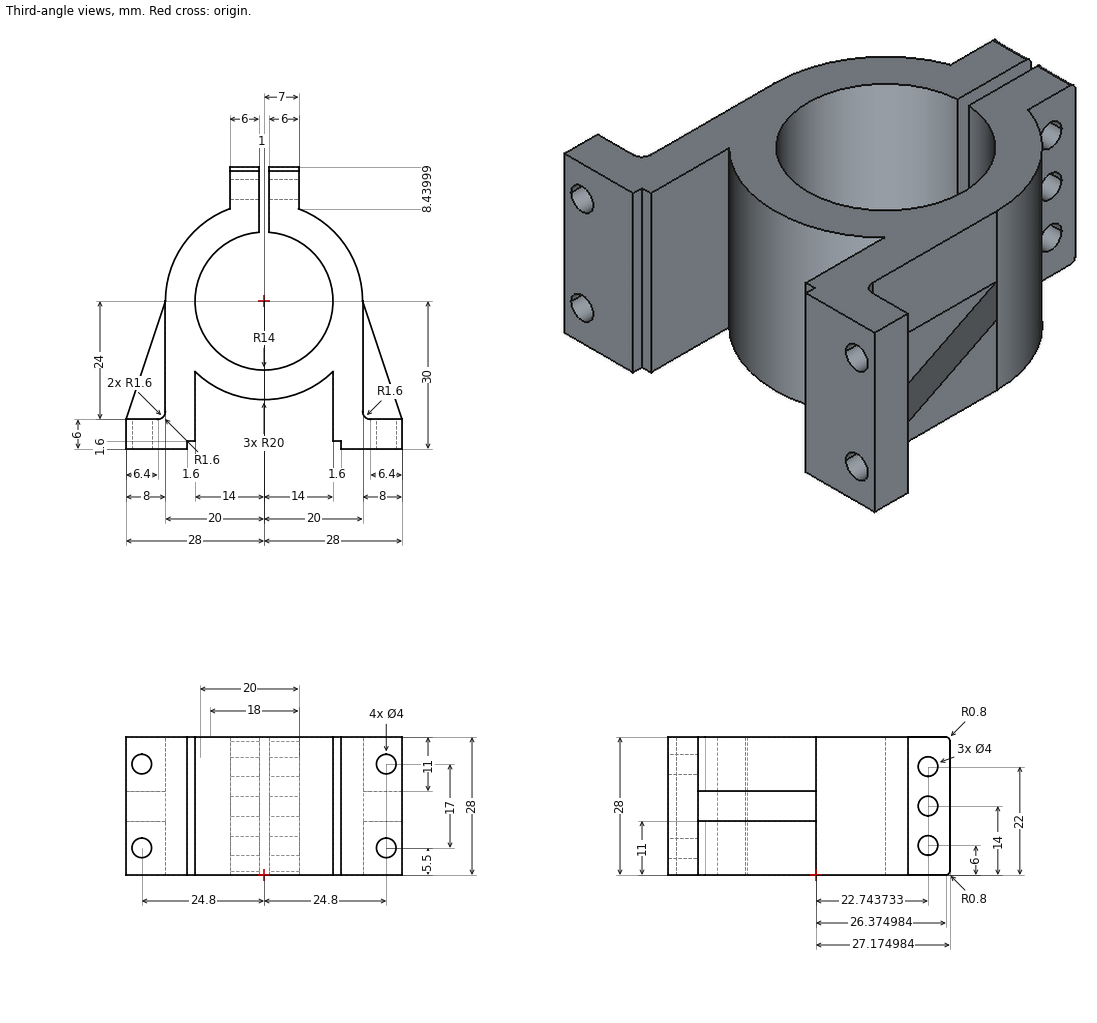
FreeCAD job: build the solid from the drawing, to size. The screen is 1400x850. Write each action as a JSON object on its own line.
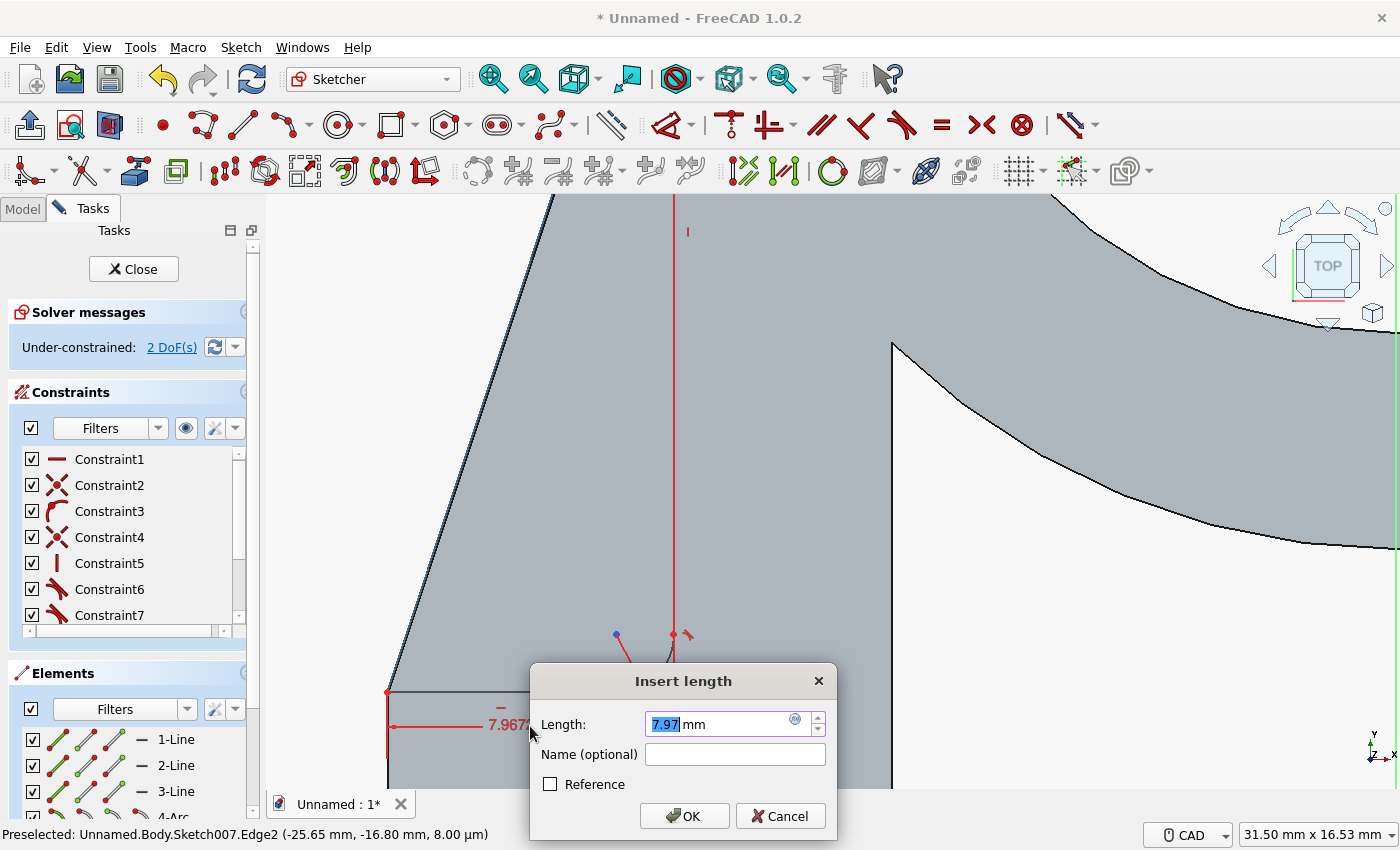
{"action": "type", "text": "8"}
{"action": "key", "text": "Return"}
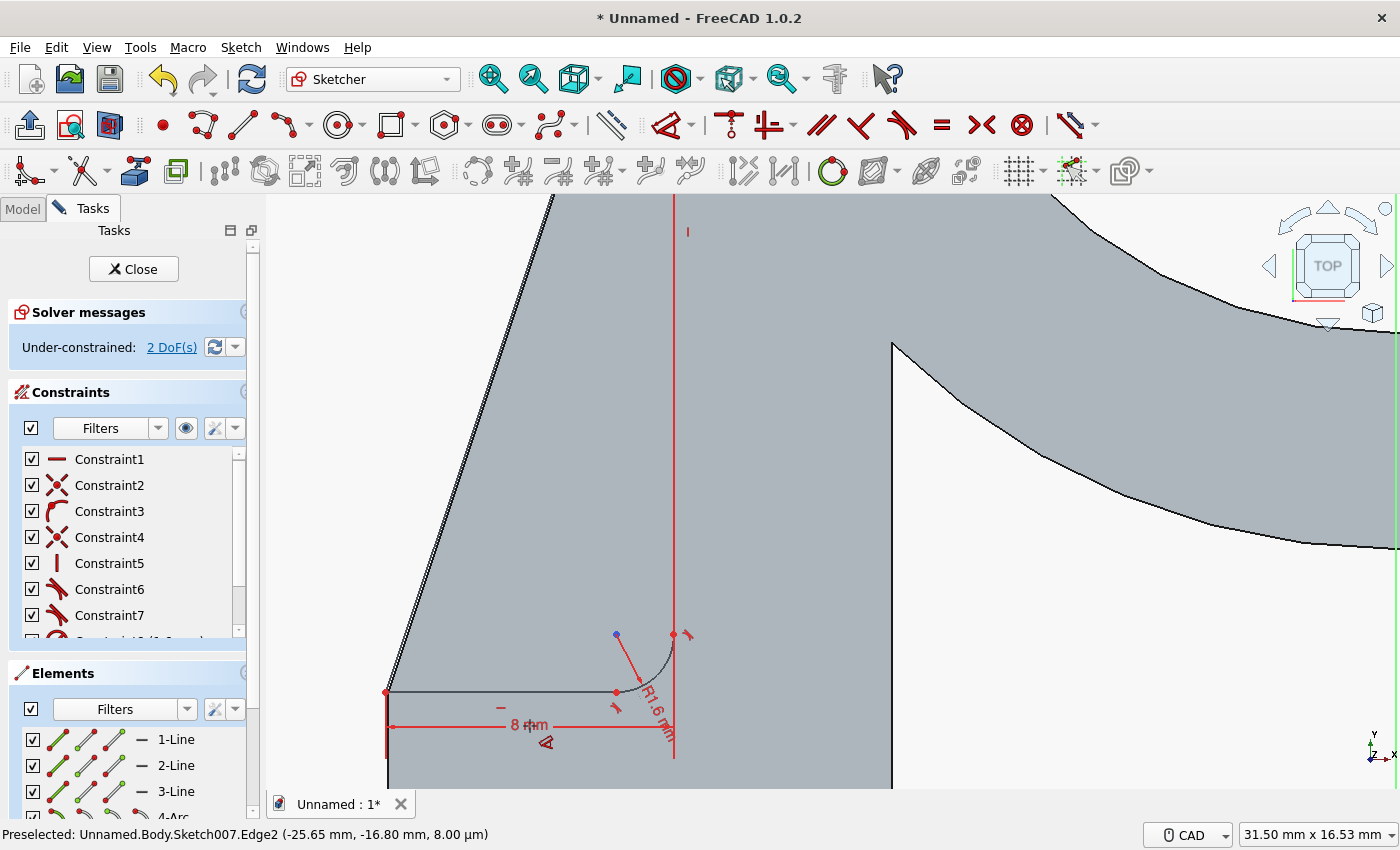
{"action": "left_click", "coordinate": [616, 692]}
{"action": "left_click", "coordinate": [582, 457]}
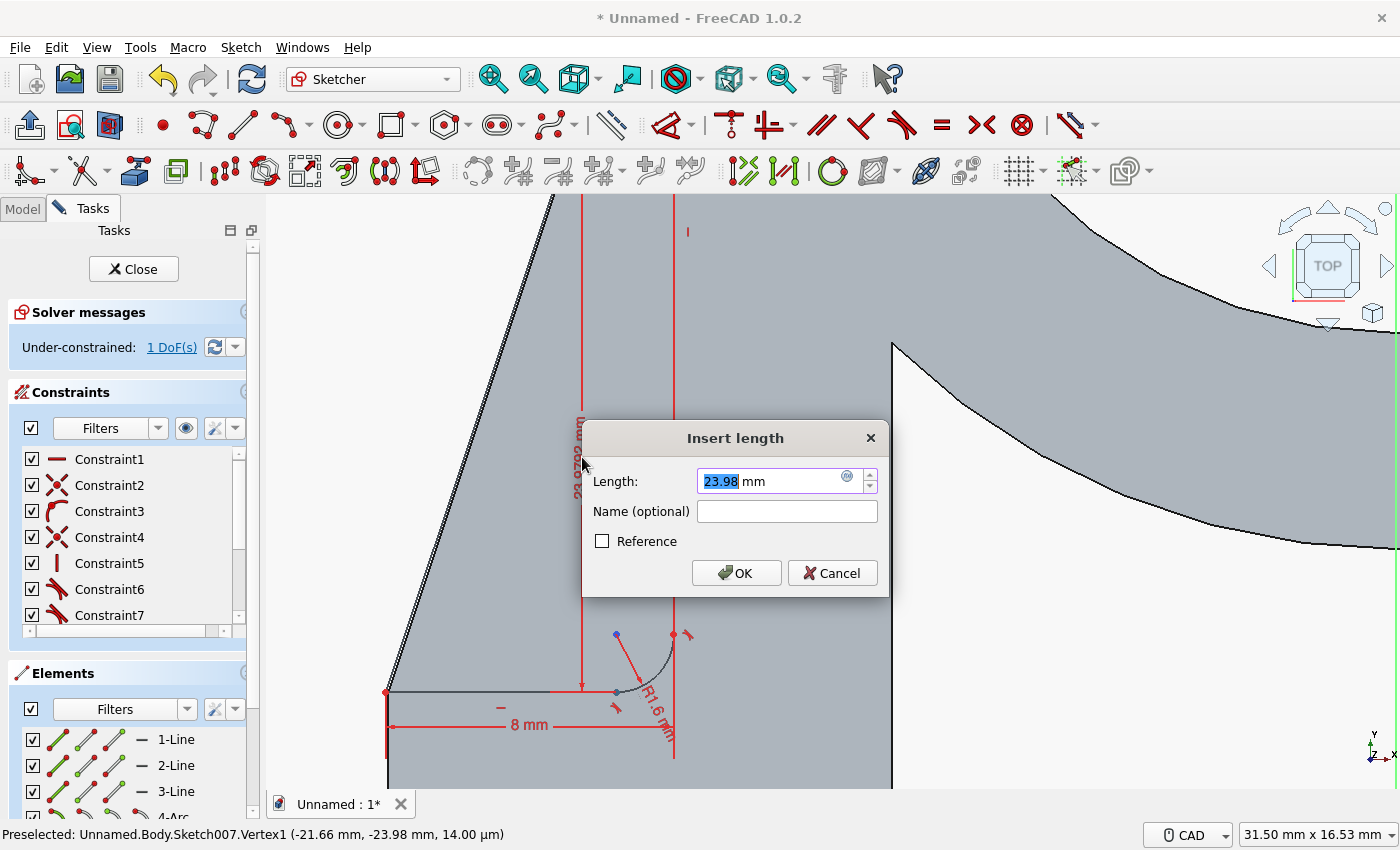
{"action": "type", "text": "24"}
{"action": "key", "text": "Return"}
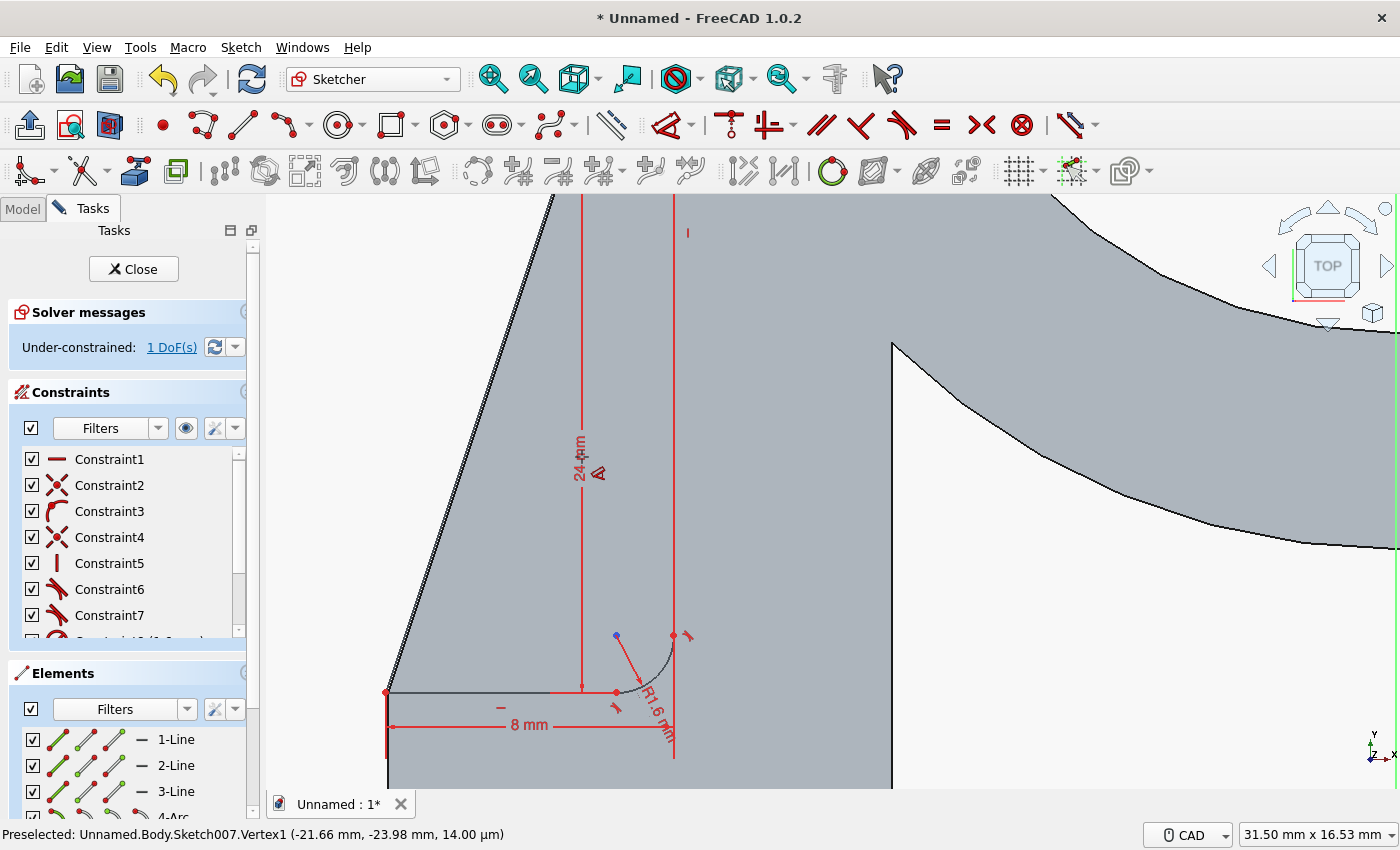
{"action": "left_click", "coordinate": [386, 693]}
{"action": "left_click", "coordinate": [810, 727]}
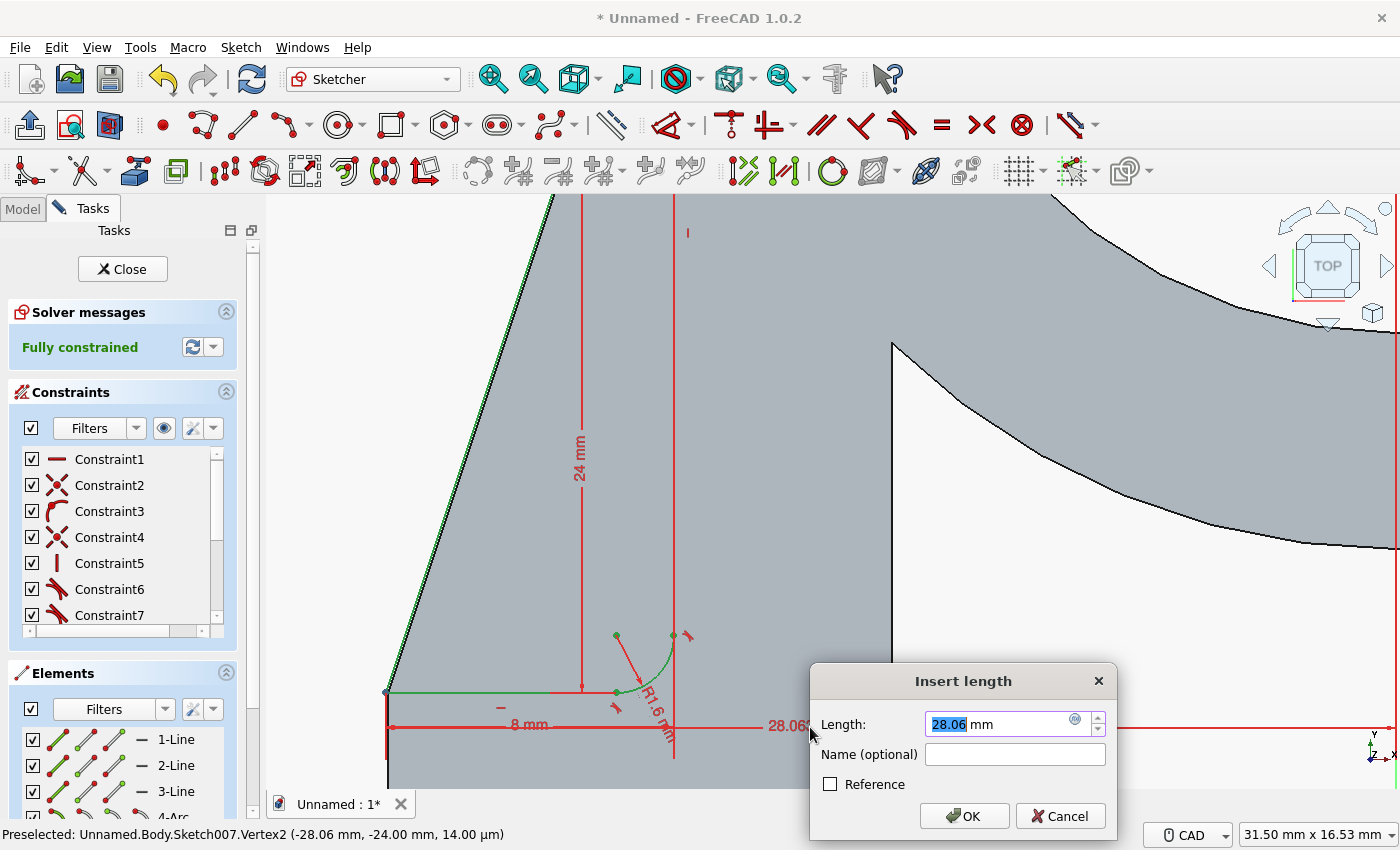
{"action": "type", "text": "28"}
{"action": "key", "text": "Return"}
{"action": "key", "text": "Escape"}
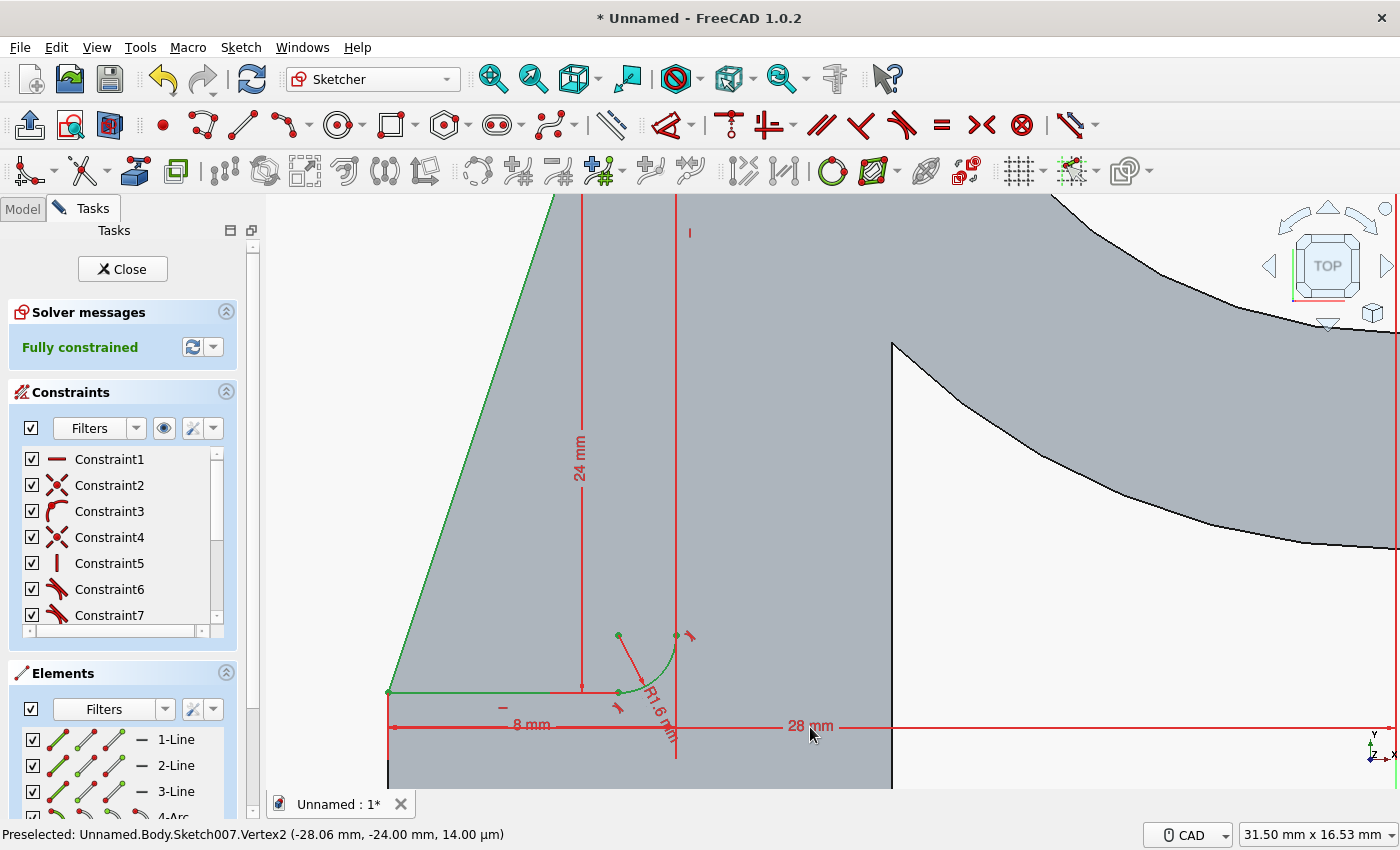
{"action": "left_click", "coordinate": [123, 269]}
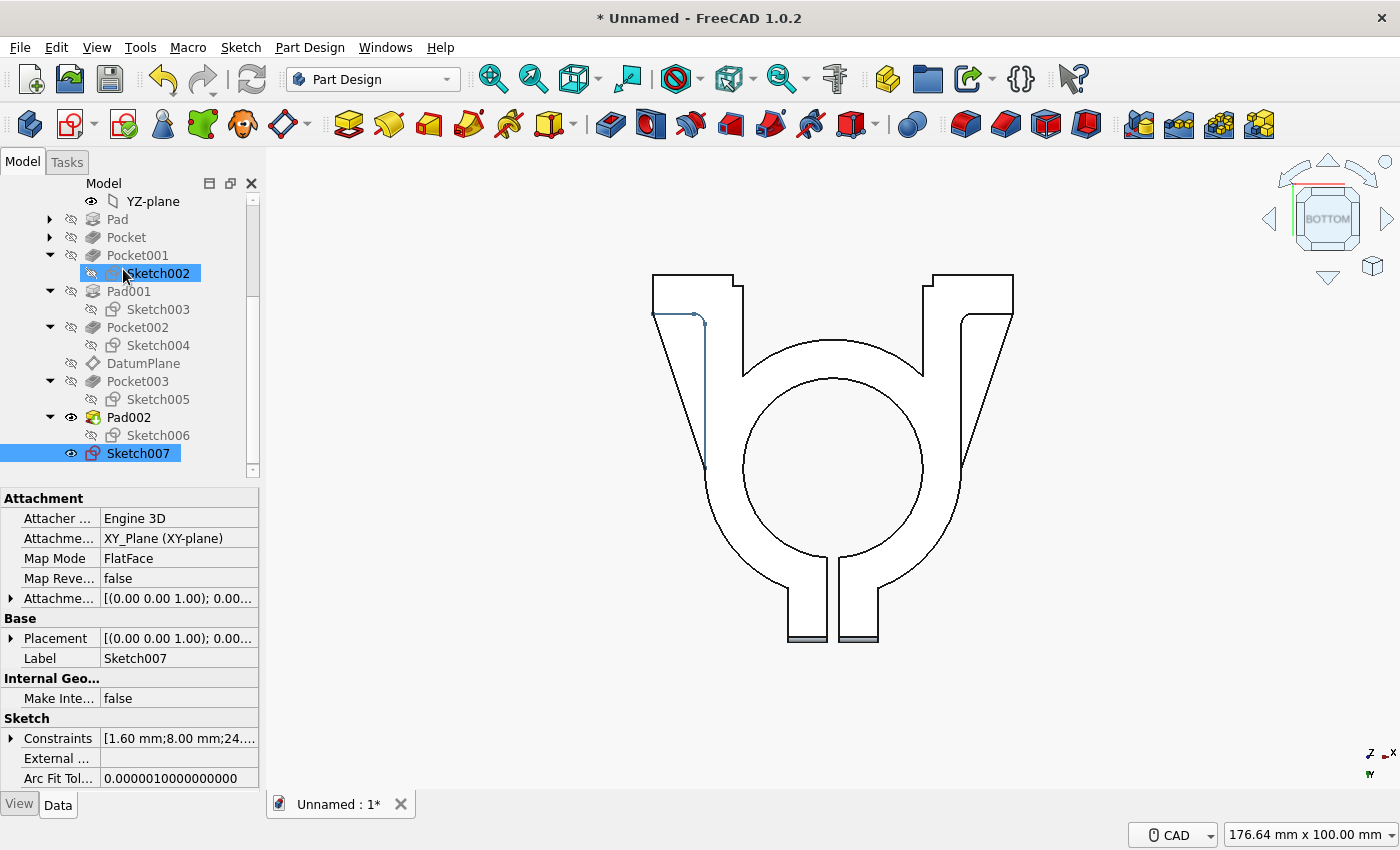
{"action": "left_click", "coordinate": [612, 124]}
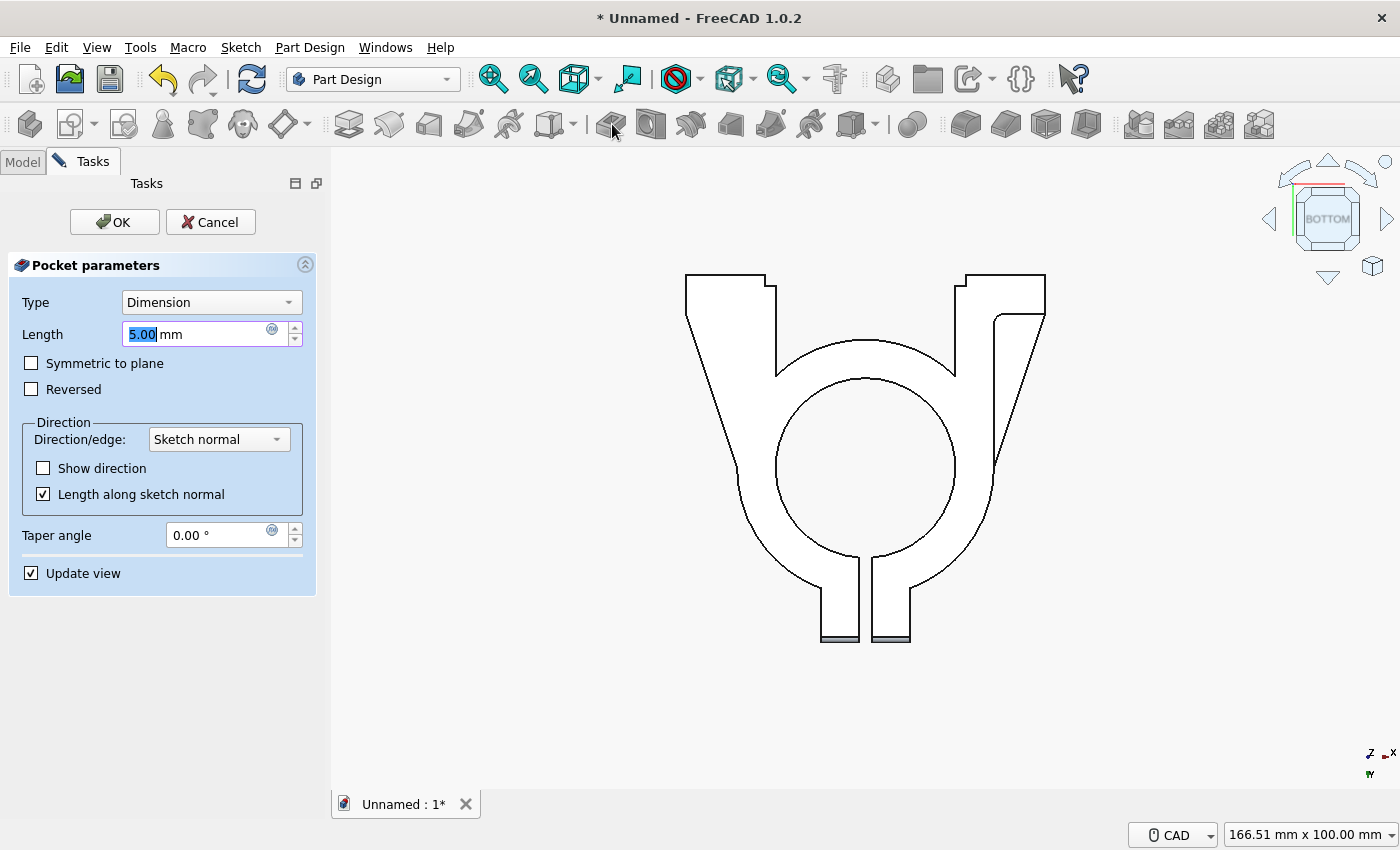
{"action": "type", "text": "11"}
{"action": "key", "text": "Tab"}